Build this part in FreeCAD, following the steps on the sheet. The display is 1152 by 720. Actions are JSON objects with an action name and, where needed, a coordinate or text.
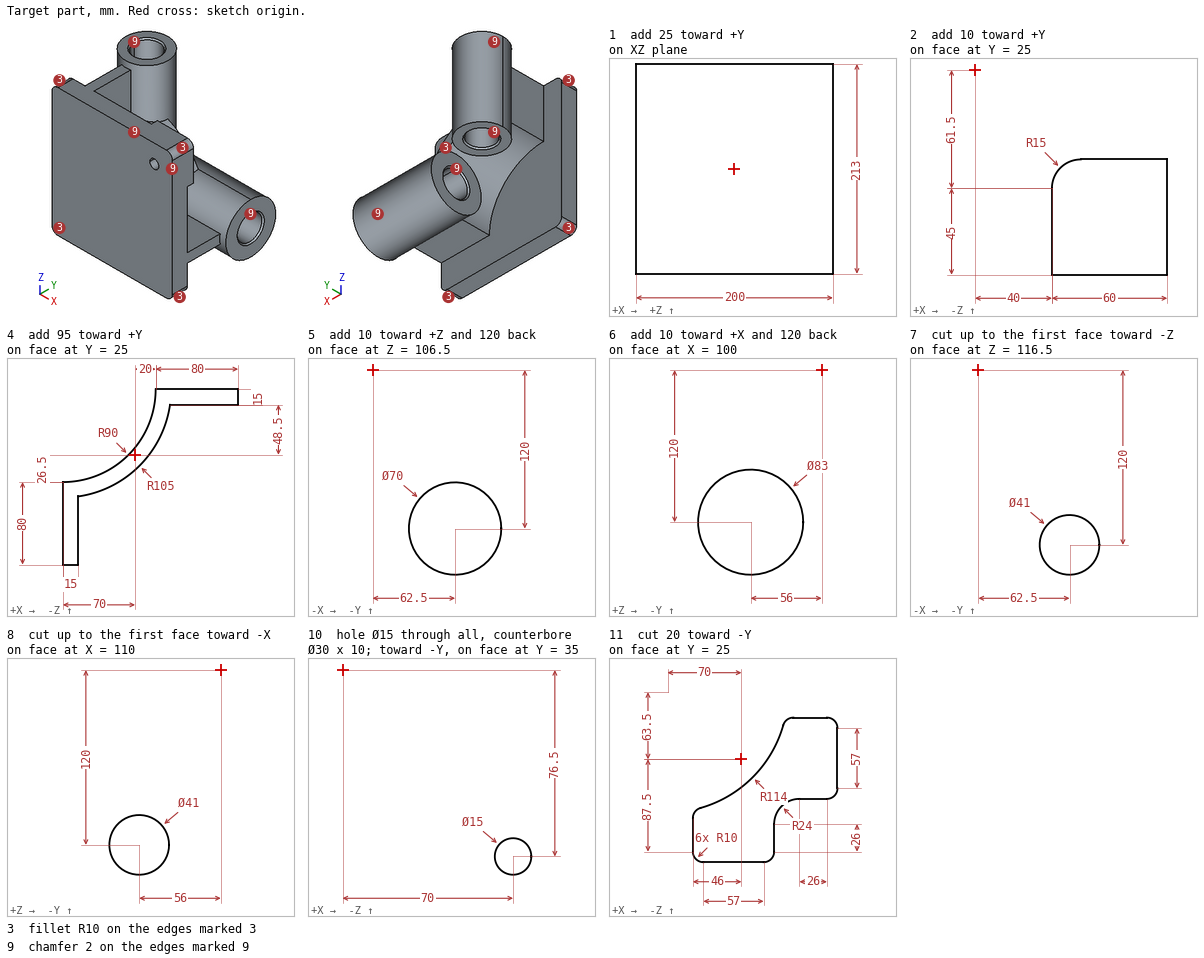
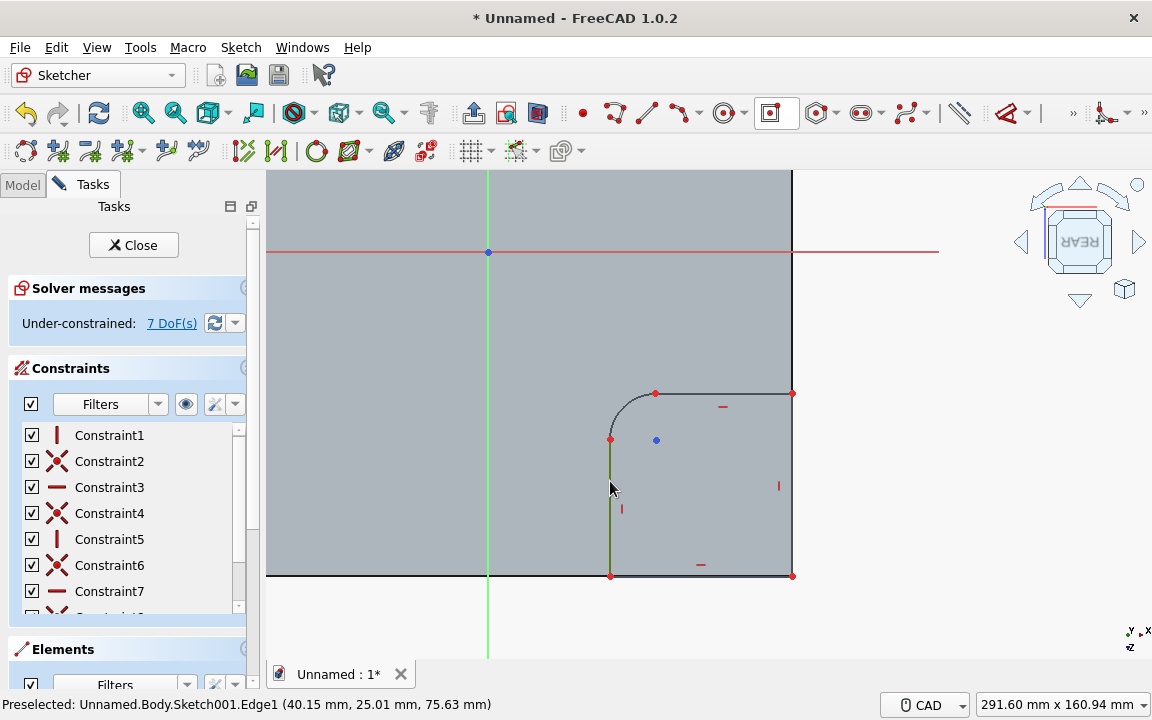
{"action": "left_click", "coordinate": [635, 399]}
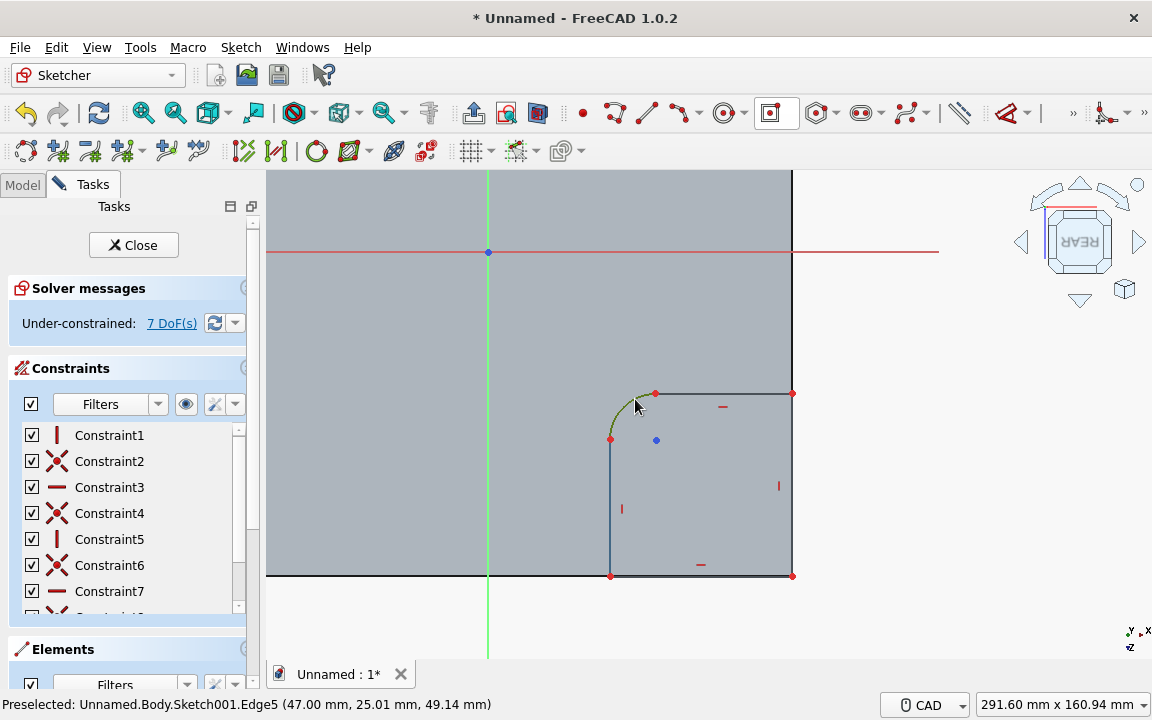
{"action": "key", "text": "t"}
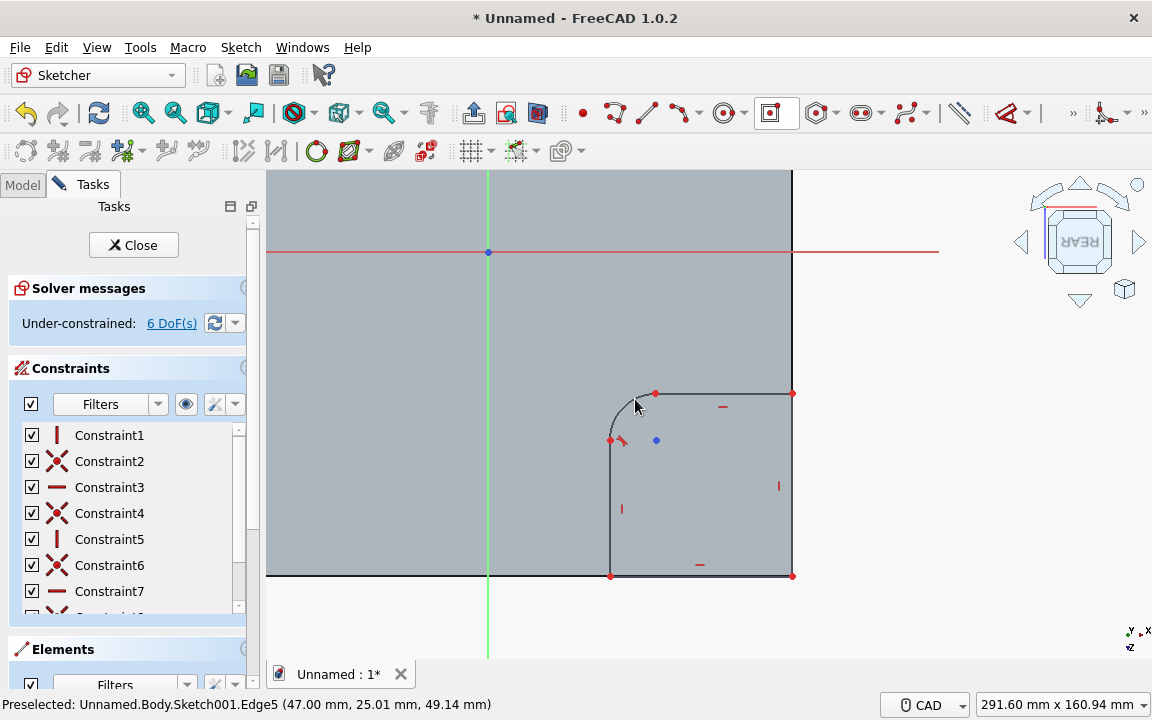
{"action": "left_click", "coordinate": [751, 394]}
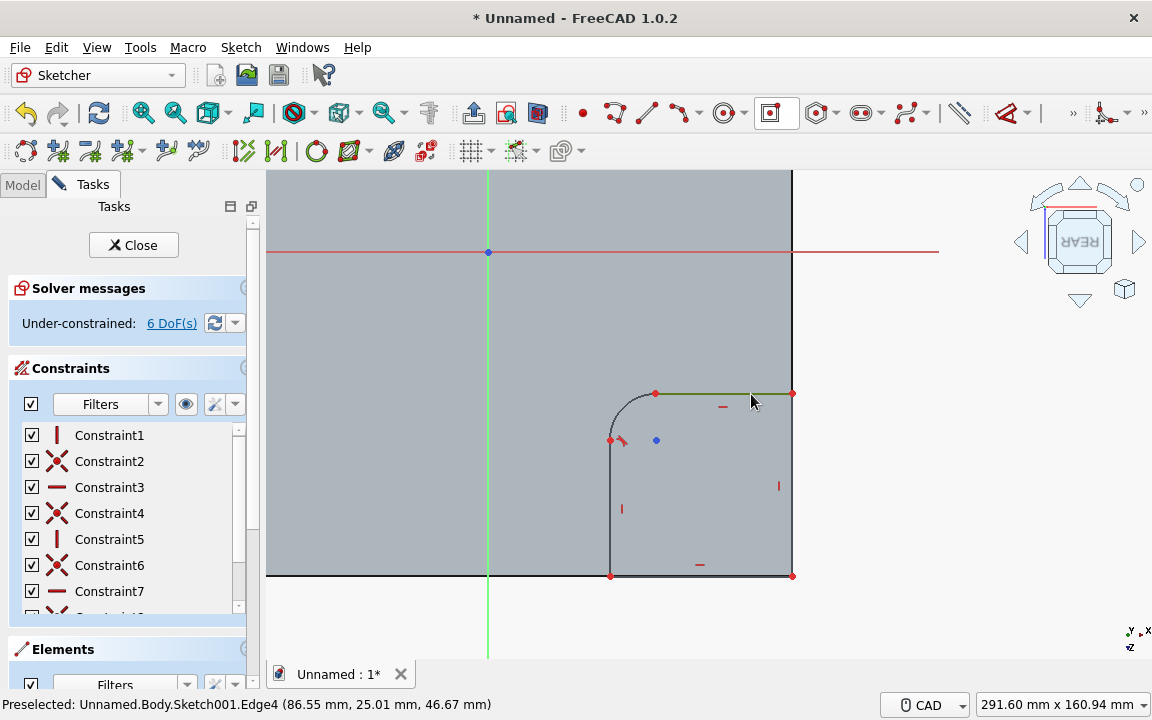
{"action": "left_click", "coordinate": [634, 399]}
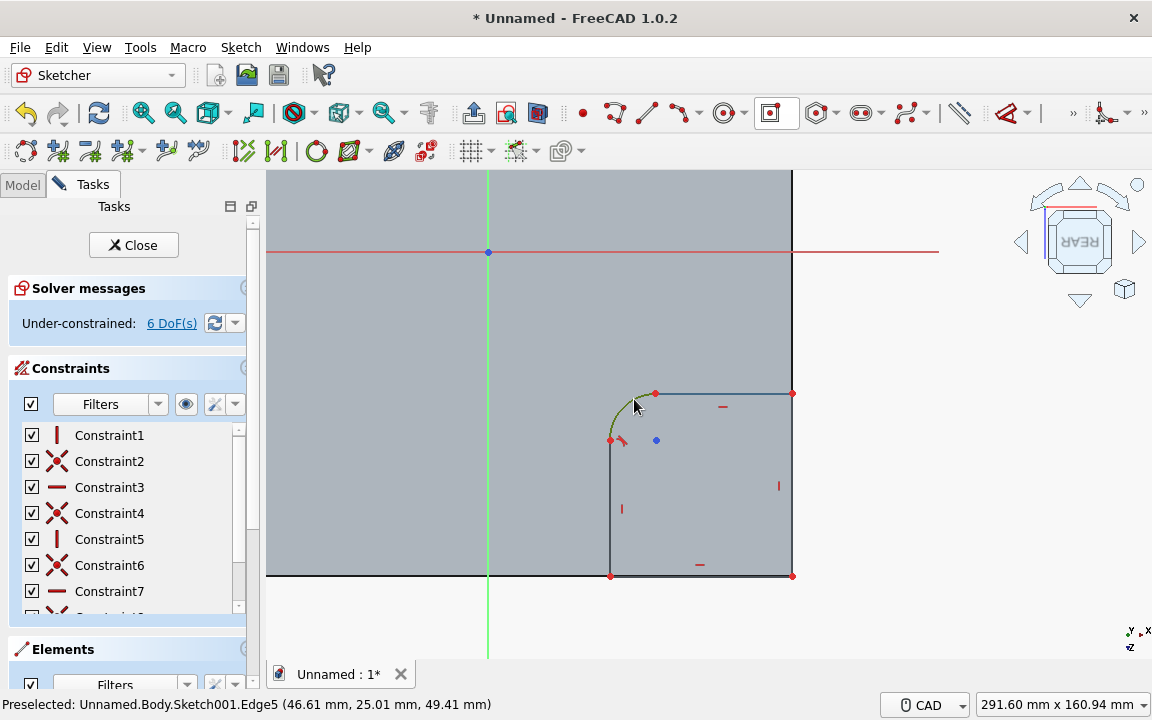
{"action": "key", "text": "t"}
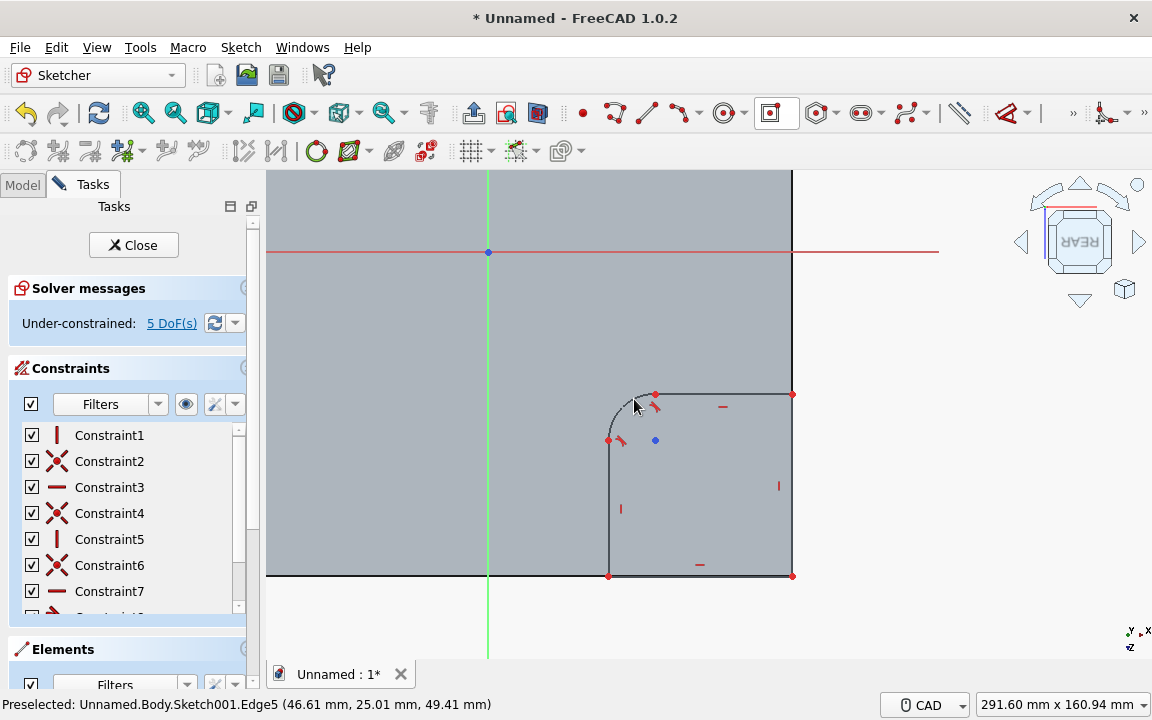
{"action": "left_click", "coordinate": [634, 399]}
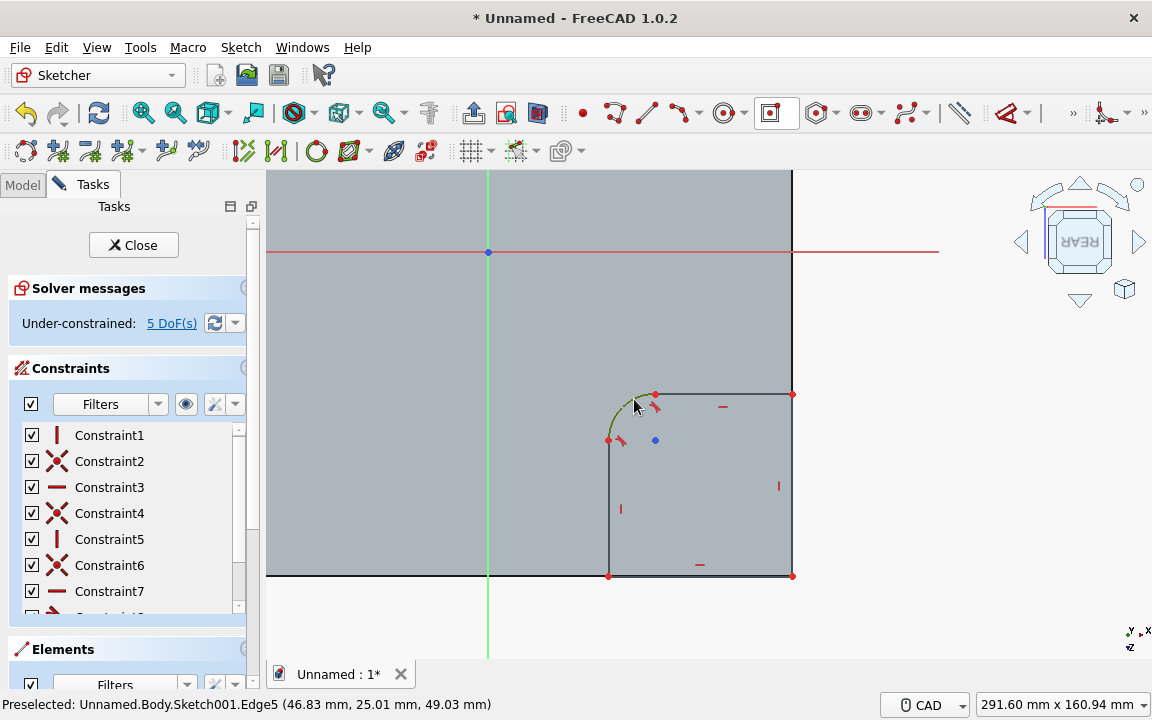
{"action": "key", "text": "k r"}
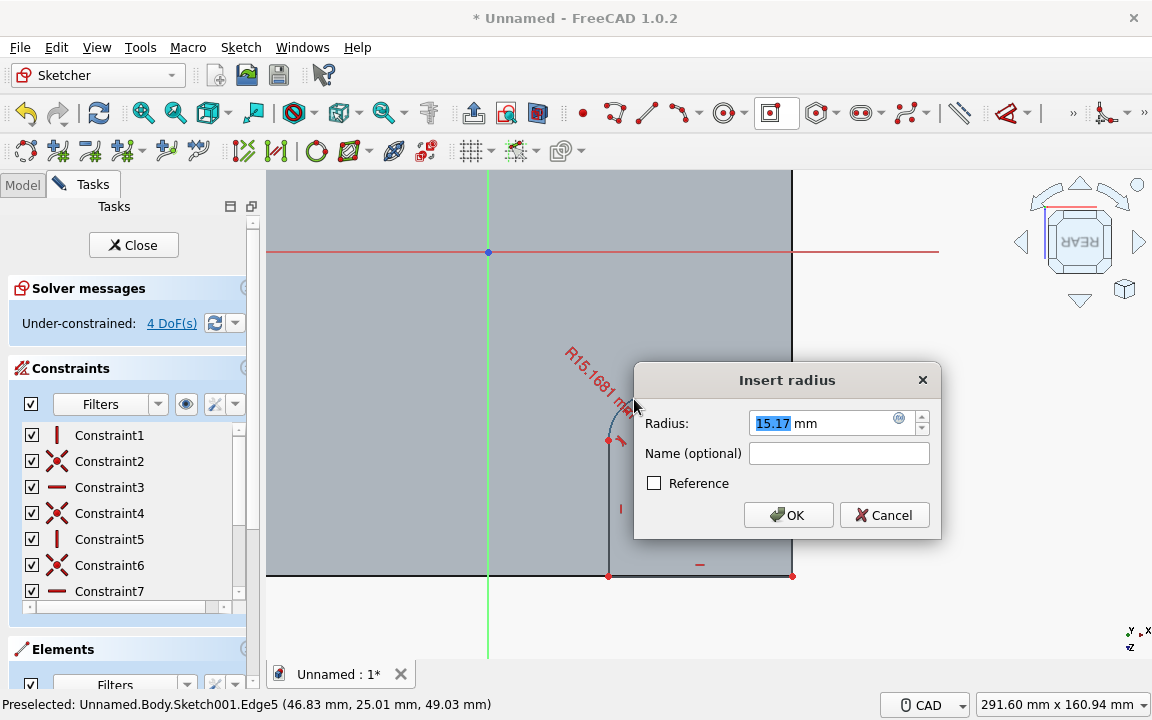
{"action": "type", "text": "15"}
{"action": "key", "text": "Return"}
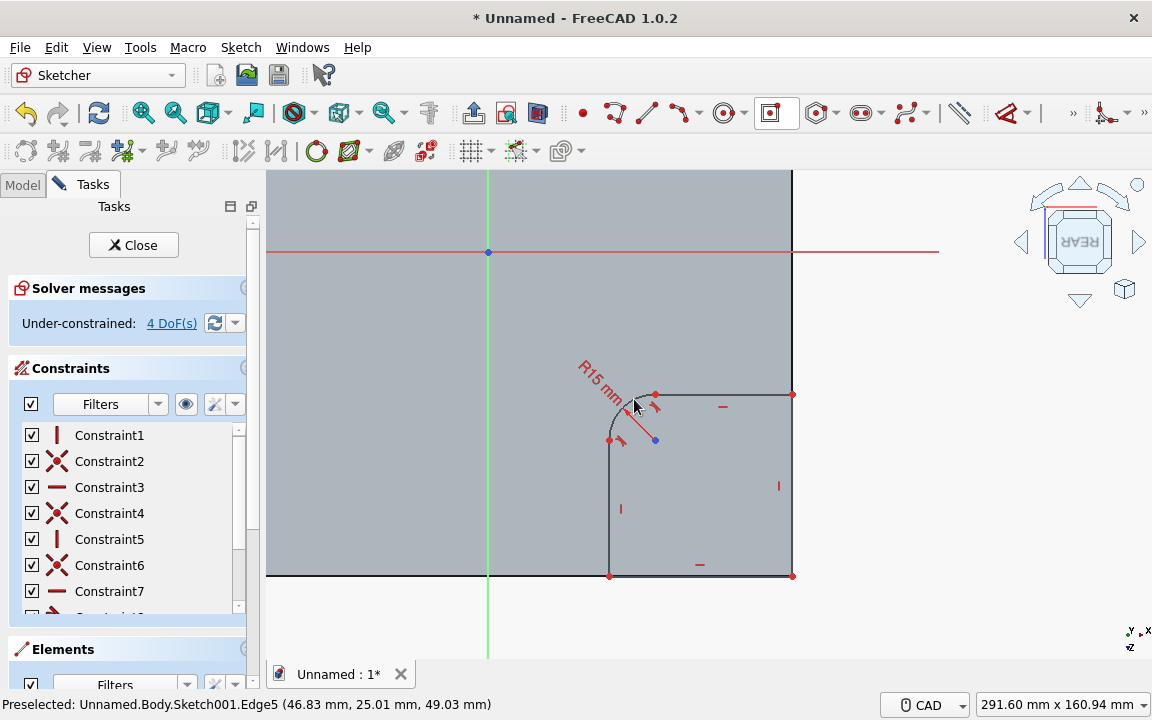
{"action": "left_click", "coordinate": [609, 481]}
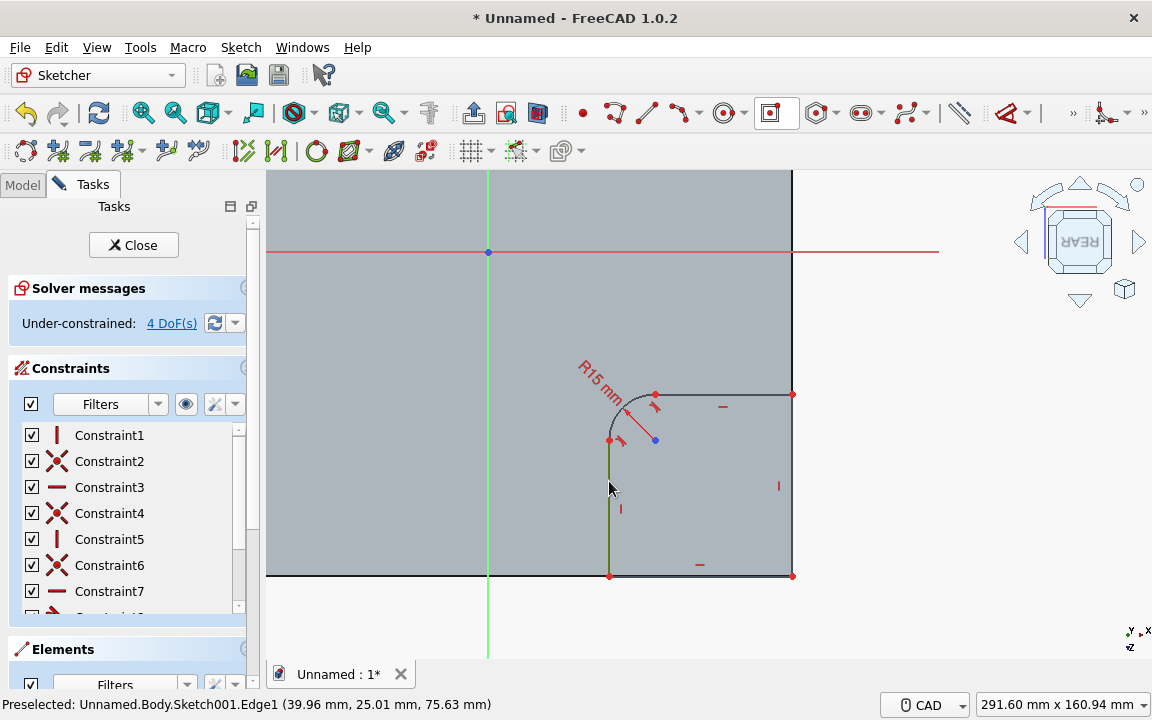
{"action": "left_click", "coordinate": [1030, 114]}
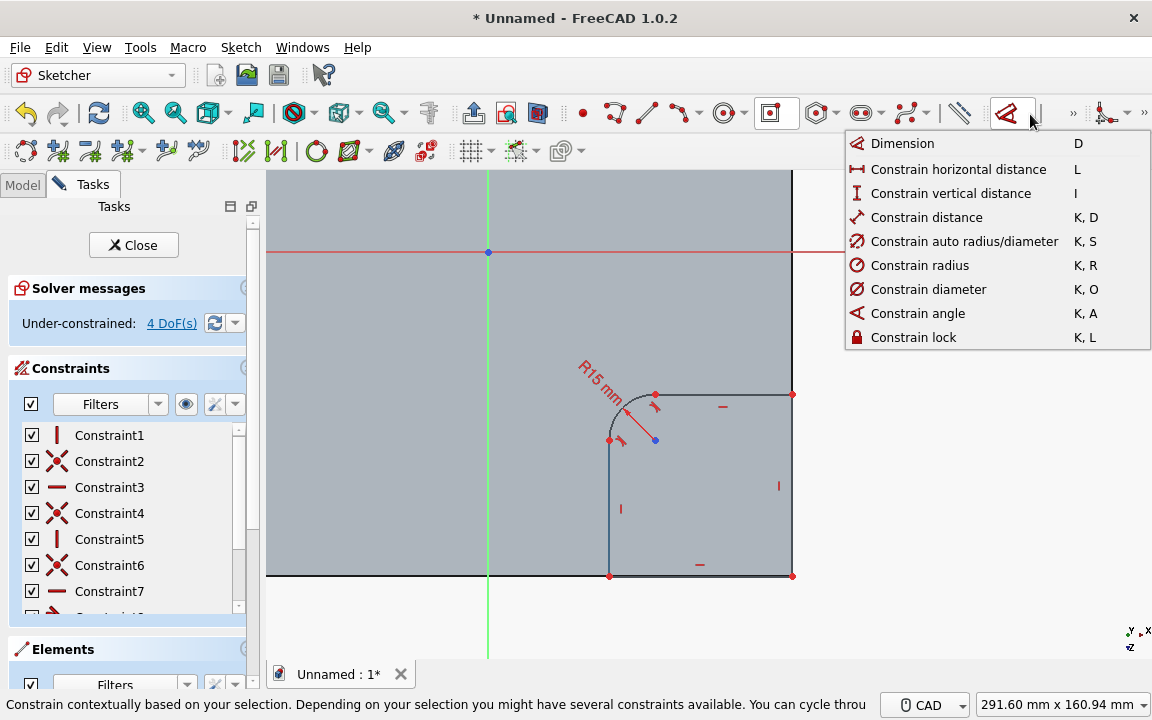
{"action": "left_click", "coordinate": [998, 193]}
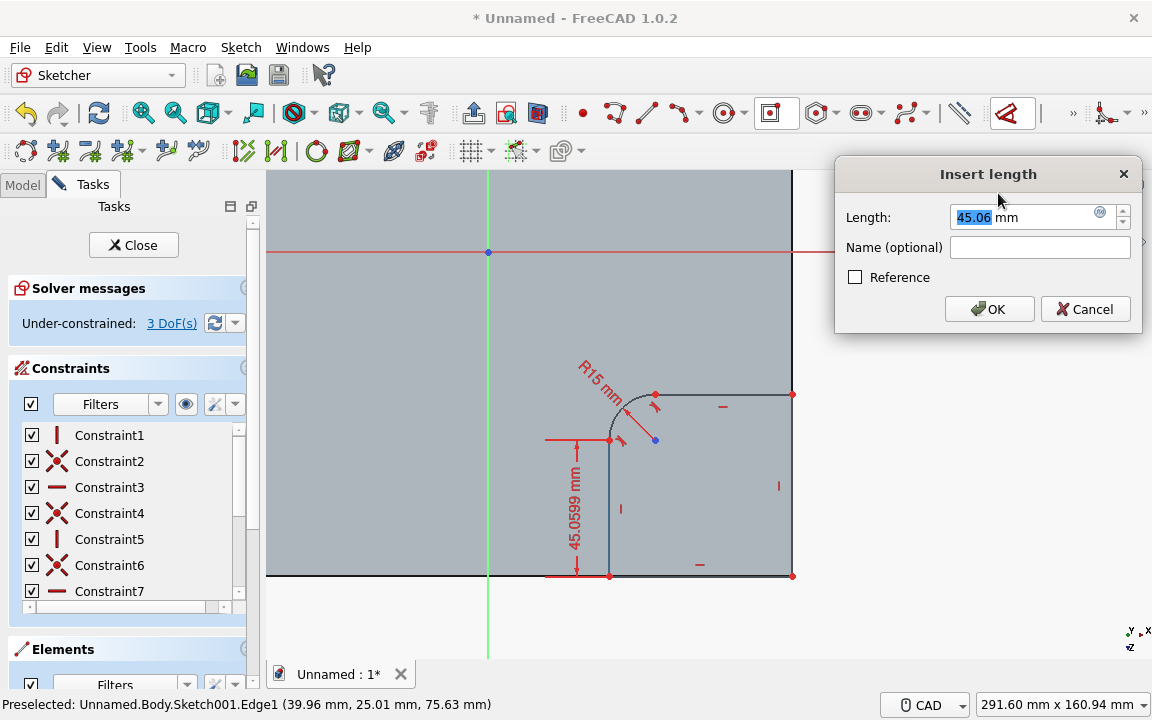
{"action": "type", "text": "45"}
{"action": "key", "text": "Return"}